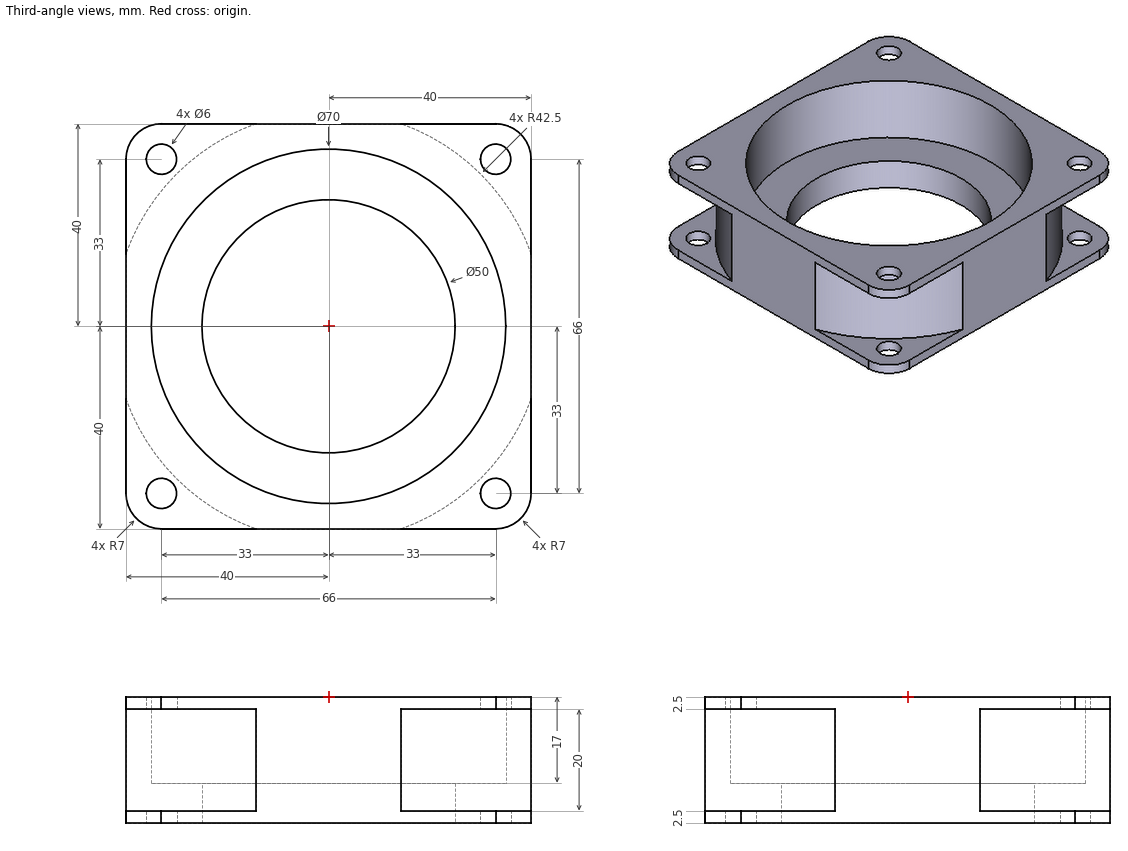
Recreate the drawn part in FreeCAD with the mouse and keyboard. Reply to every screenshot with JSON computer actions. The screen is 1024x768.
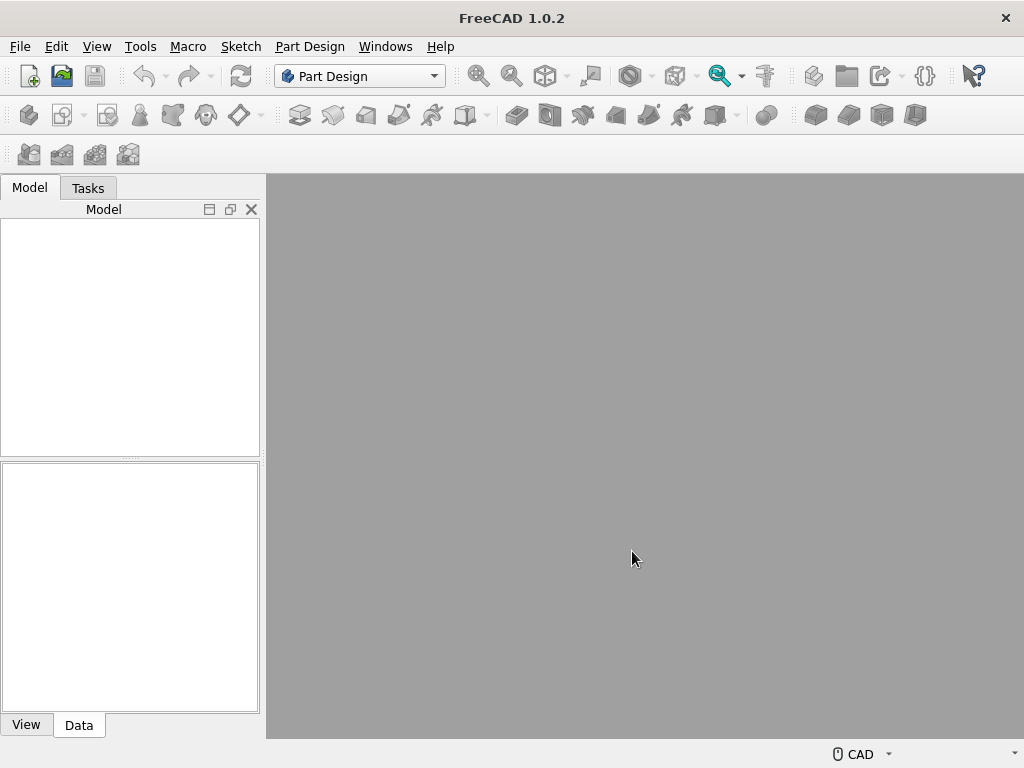
{"action": "left_click", "coordinate": [29, 76]}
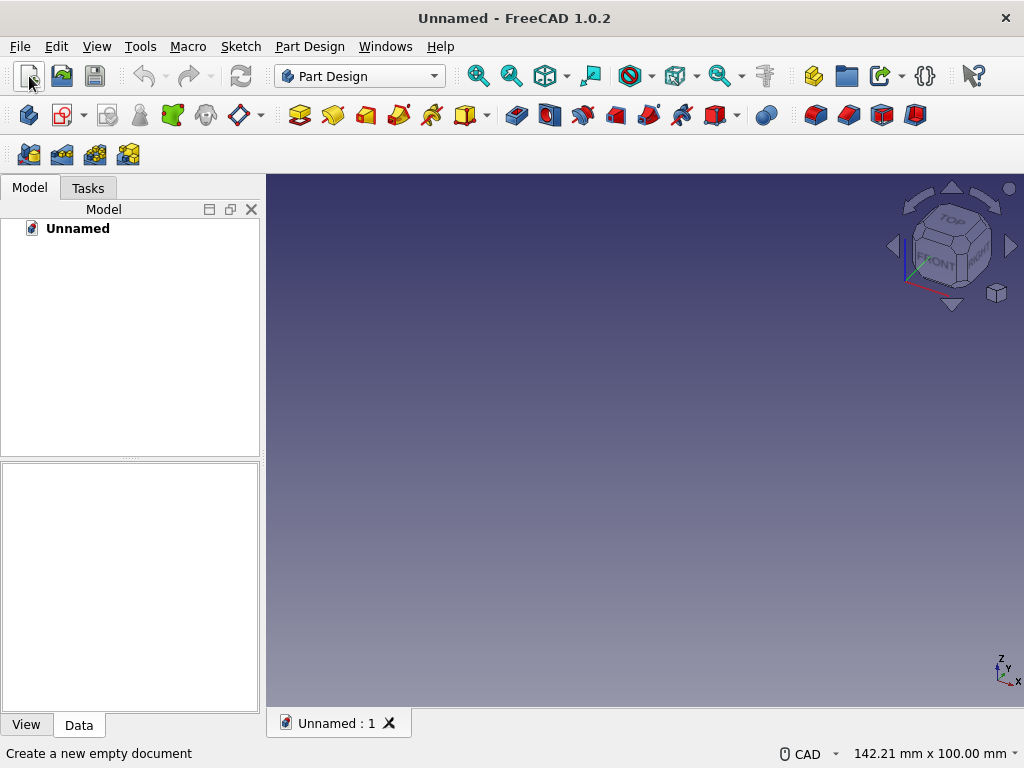
{"action": "left_click", "coordinate": [62, 116]}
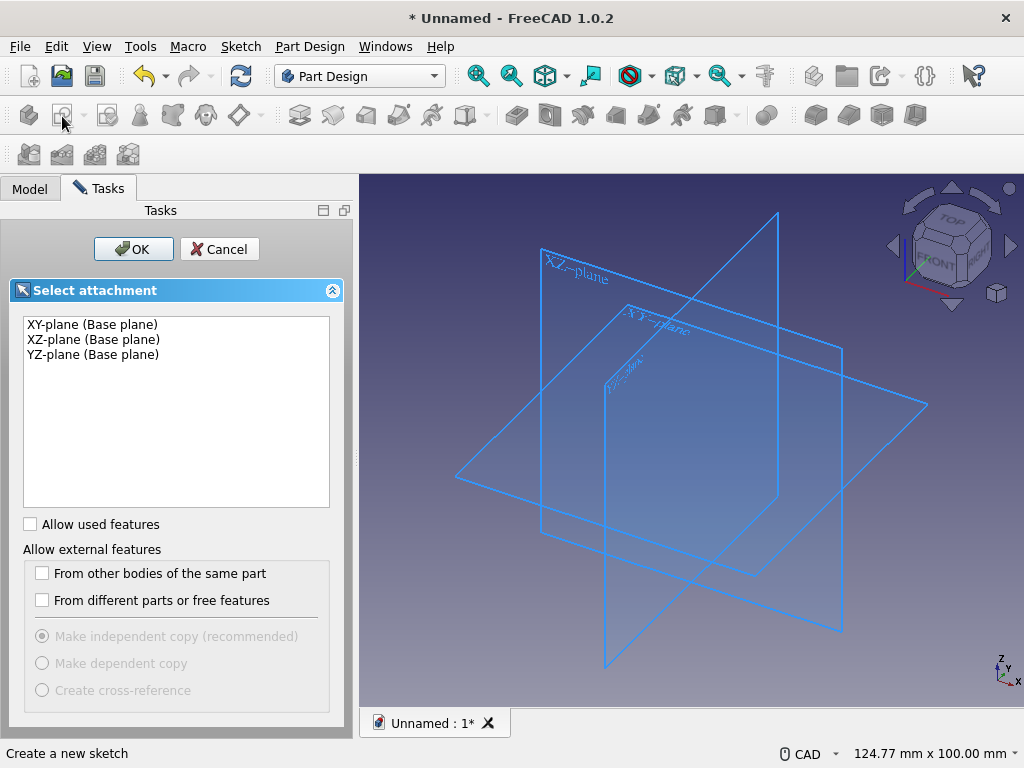
{"action": "left_click", "coordinate": [84, 324]}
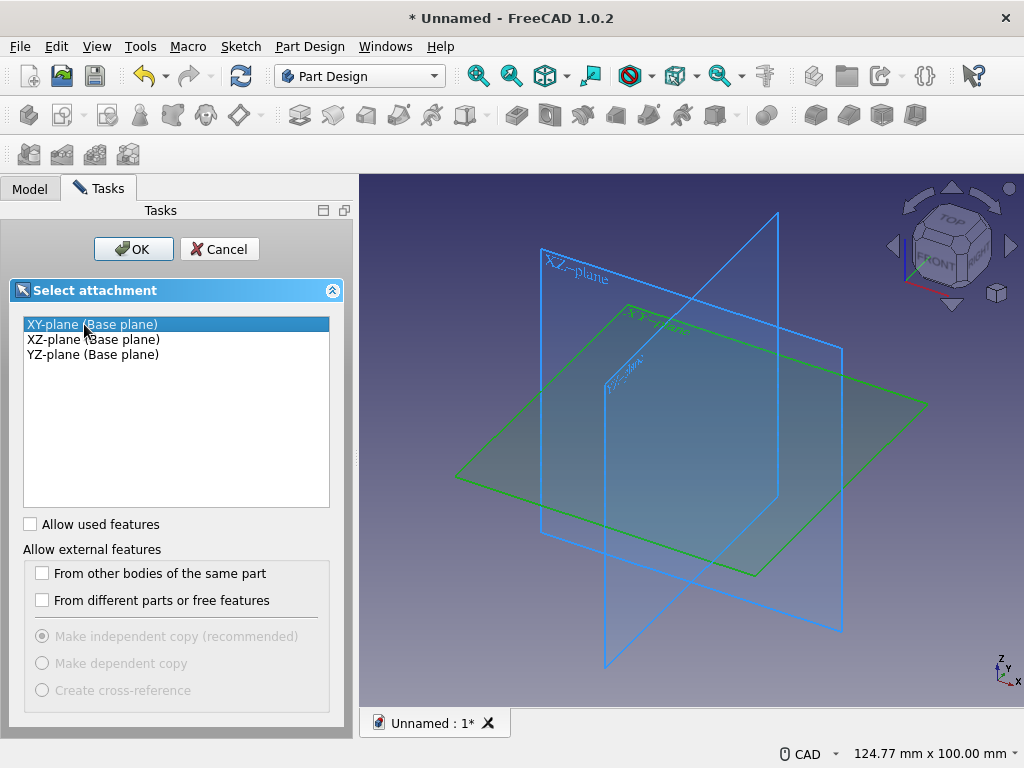
{"action": "left_click", "coordinate": [134, 249]}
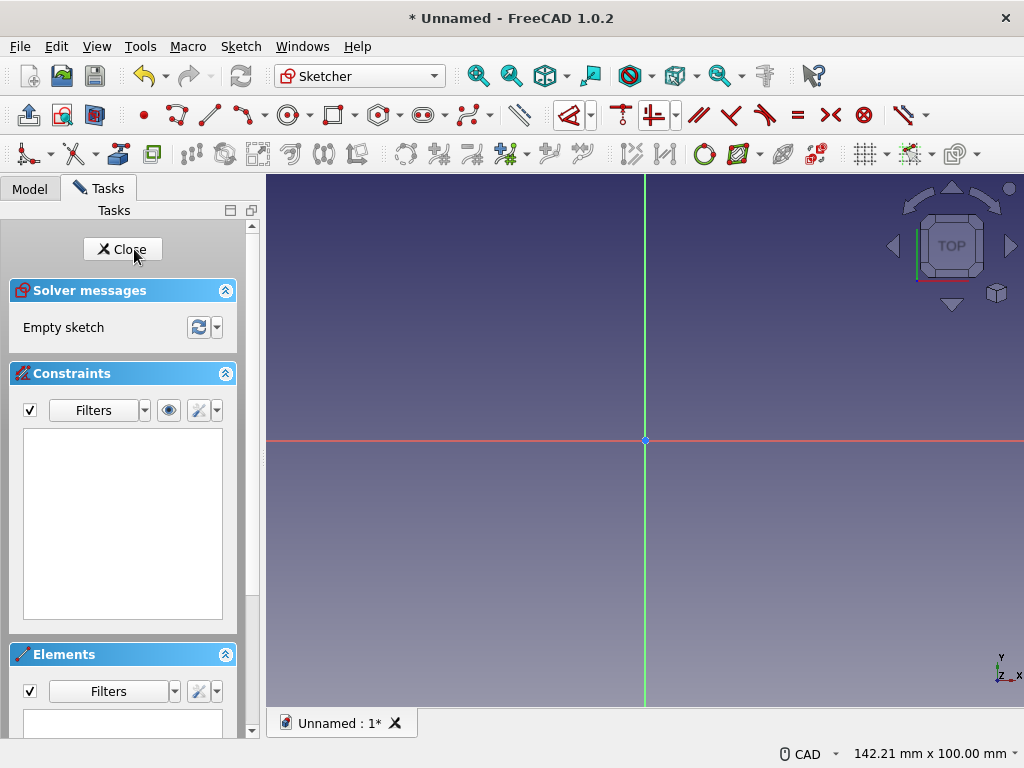
{"action": "scroll", "coordinate": [294, 440], "scroll_direction": "down", "scroll_amount": 1}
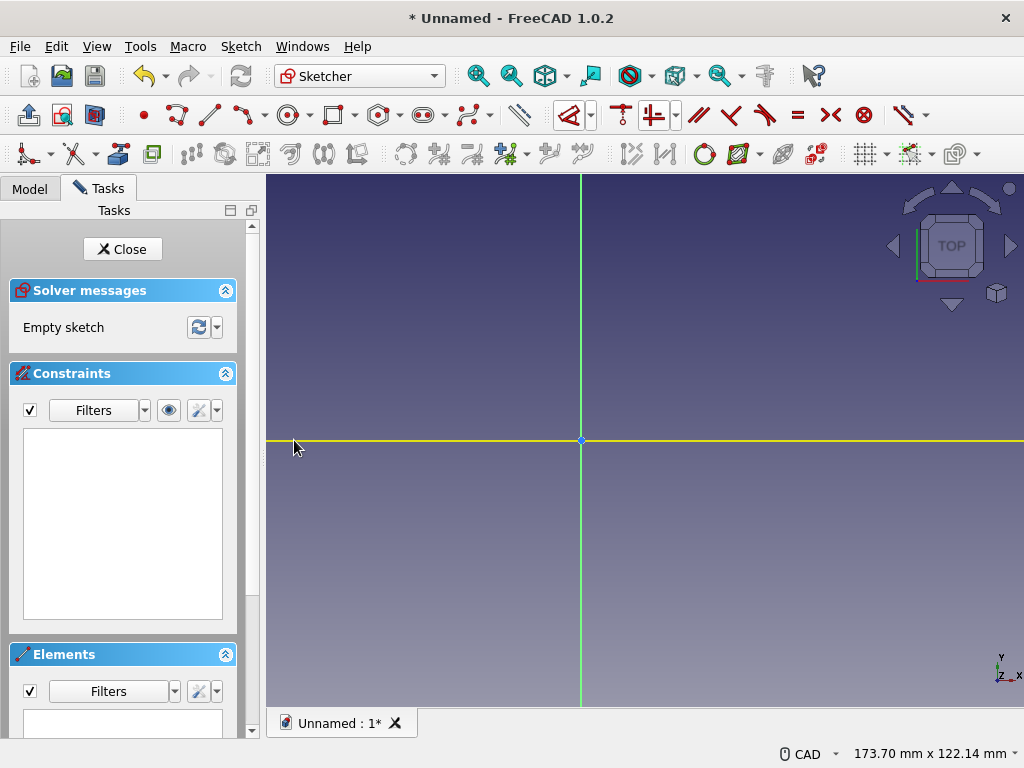
{"action": "left_click", "coordinate": [210, 116]}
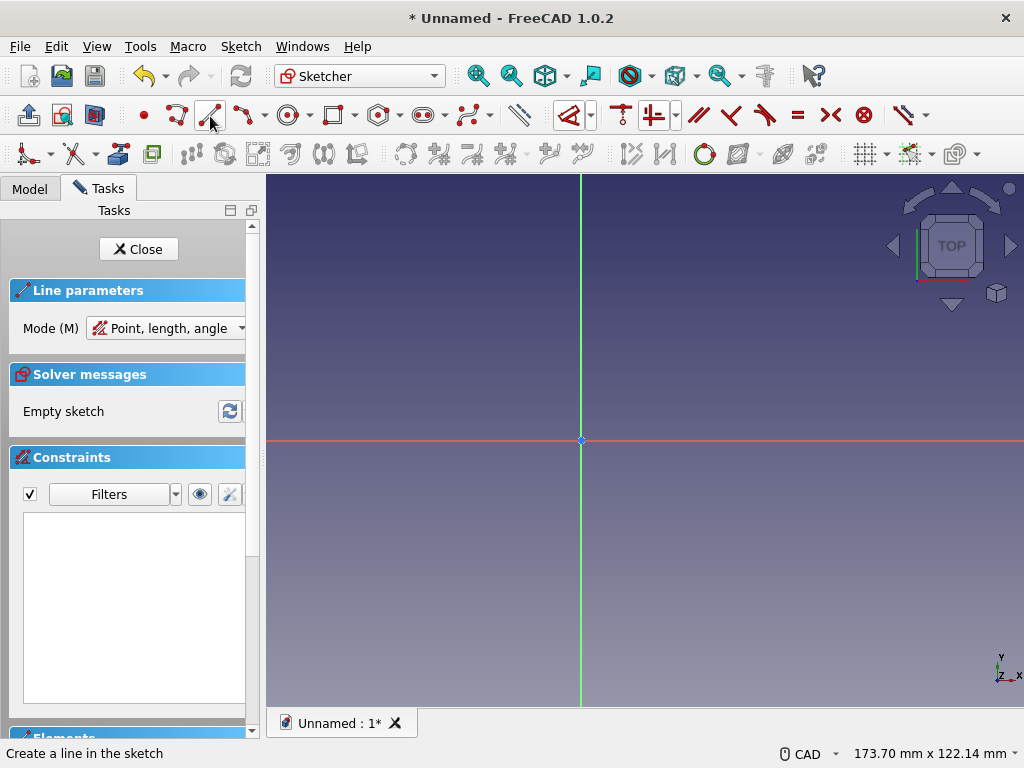
{"action": "left_click", "coordinate": [437, 615]}
{"action": "left_click", "coordinate": [725, 615]}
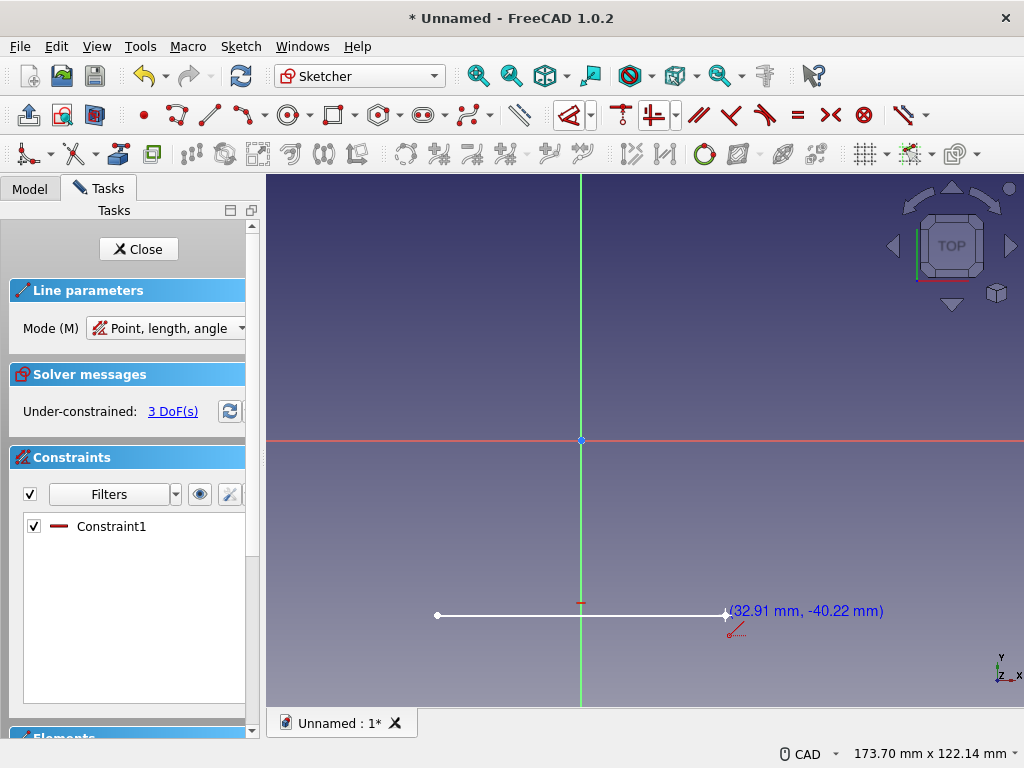
{"action": "left_click", "coordinate": [756, 585]}
{"action": "left_click", "coordinate": [756, 296]}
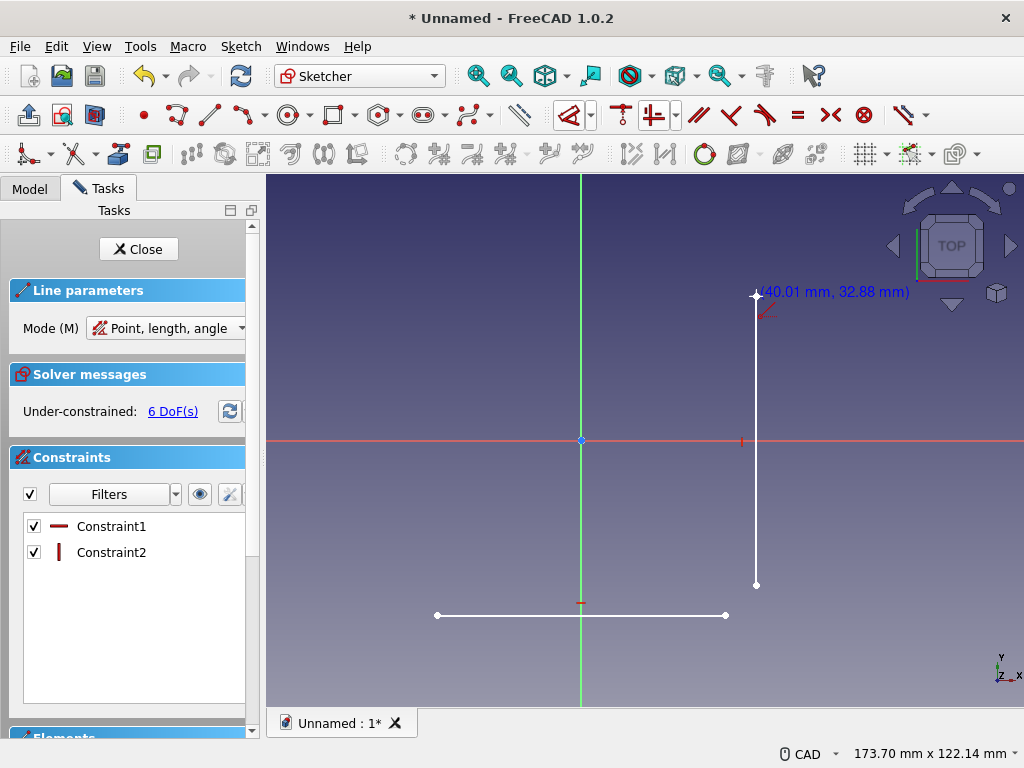
{"action": "left_click", "coordinate": [725, 266]}
{"action": "left_click", "coordinate": [437, 266]}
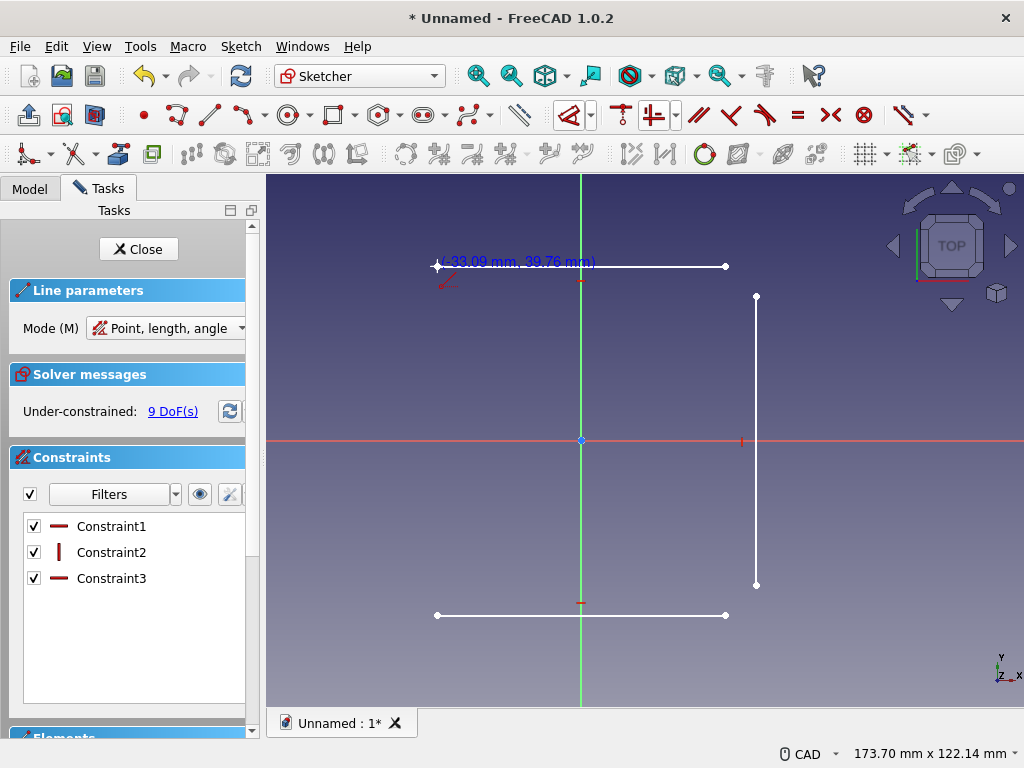
{"action": "left_click", "coordinate": [407, 296]}
{"action": "left_click", "coordinate": [407, 585]}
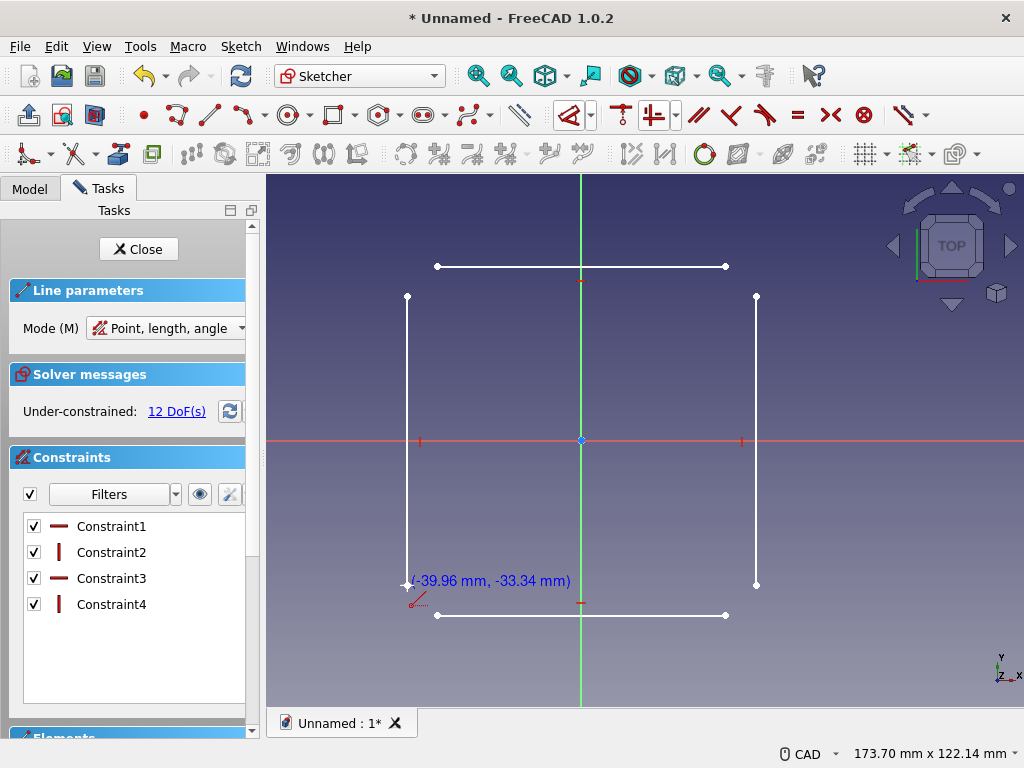
{"action": "left_click", "coordinate": [242, 116]}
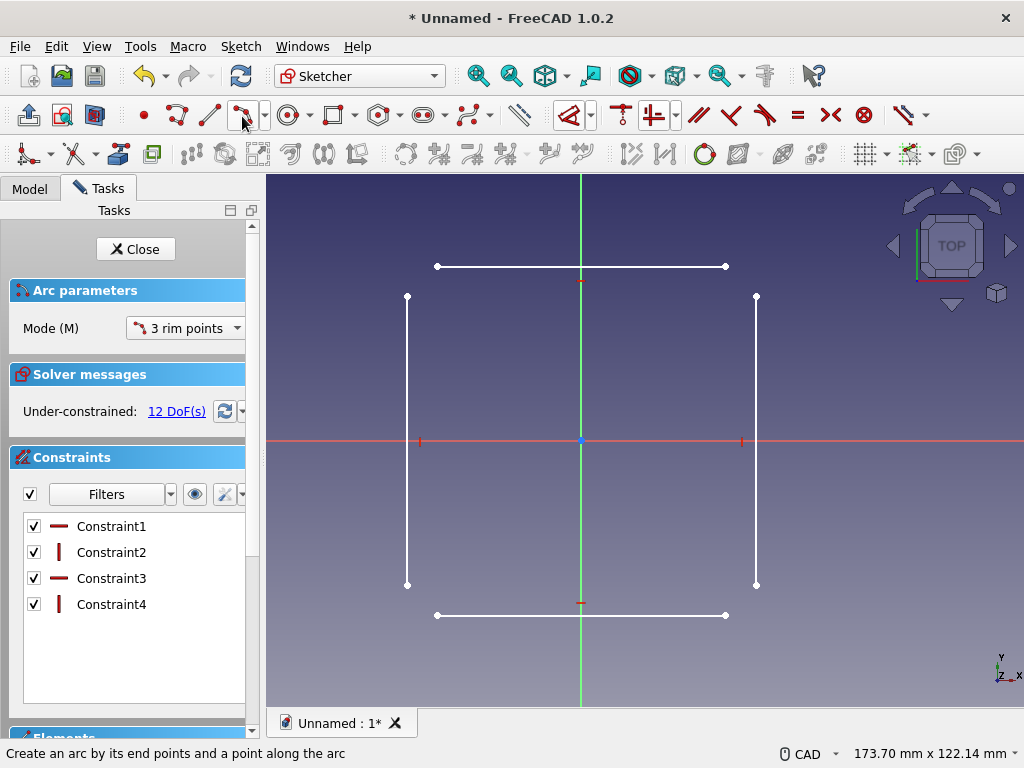
{"action": "left_click", "coordinate": [725, 616]}
{"action": "left_click", "coordinate": [756, 586]}